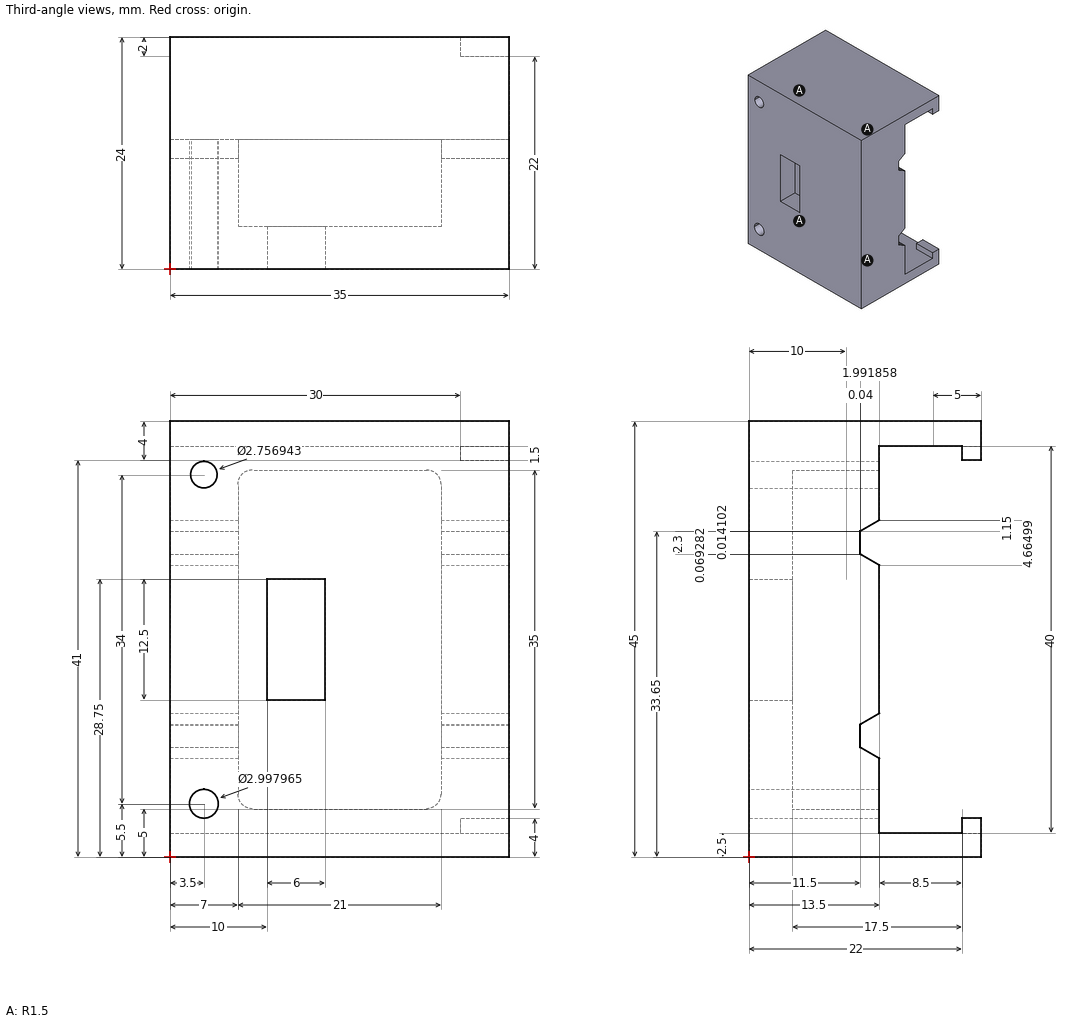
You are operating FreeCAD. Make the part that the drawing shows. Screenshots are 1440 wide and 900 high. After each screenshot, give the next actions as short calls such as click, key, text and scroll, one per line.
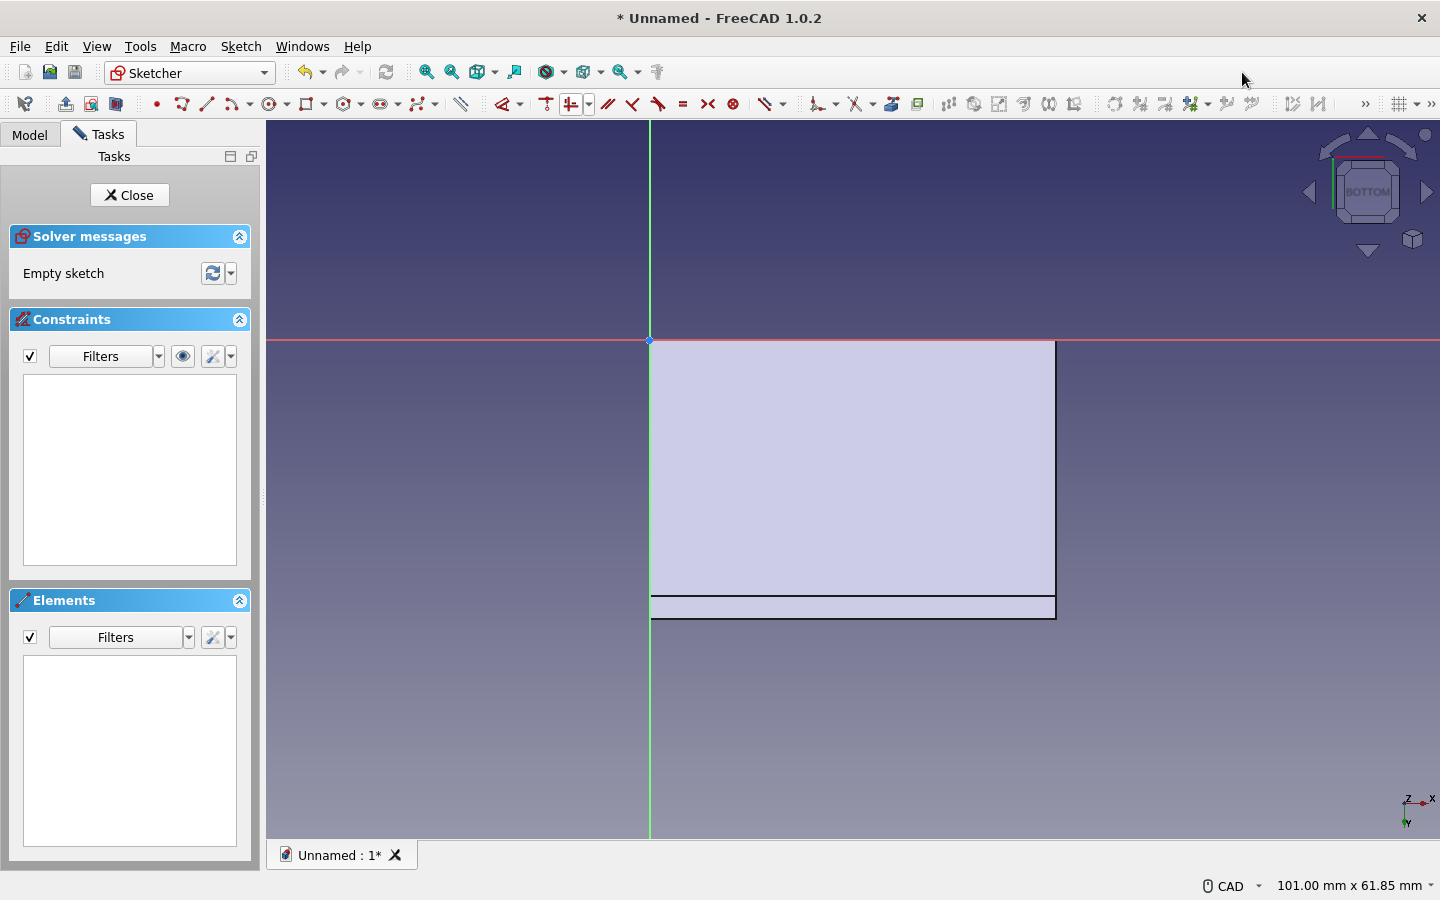
scroll(936, 480, up, 3)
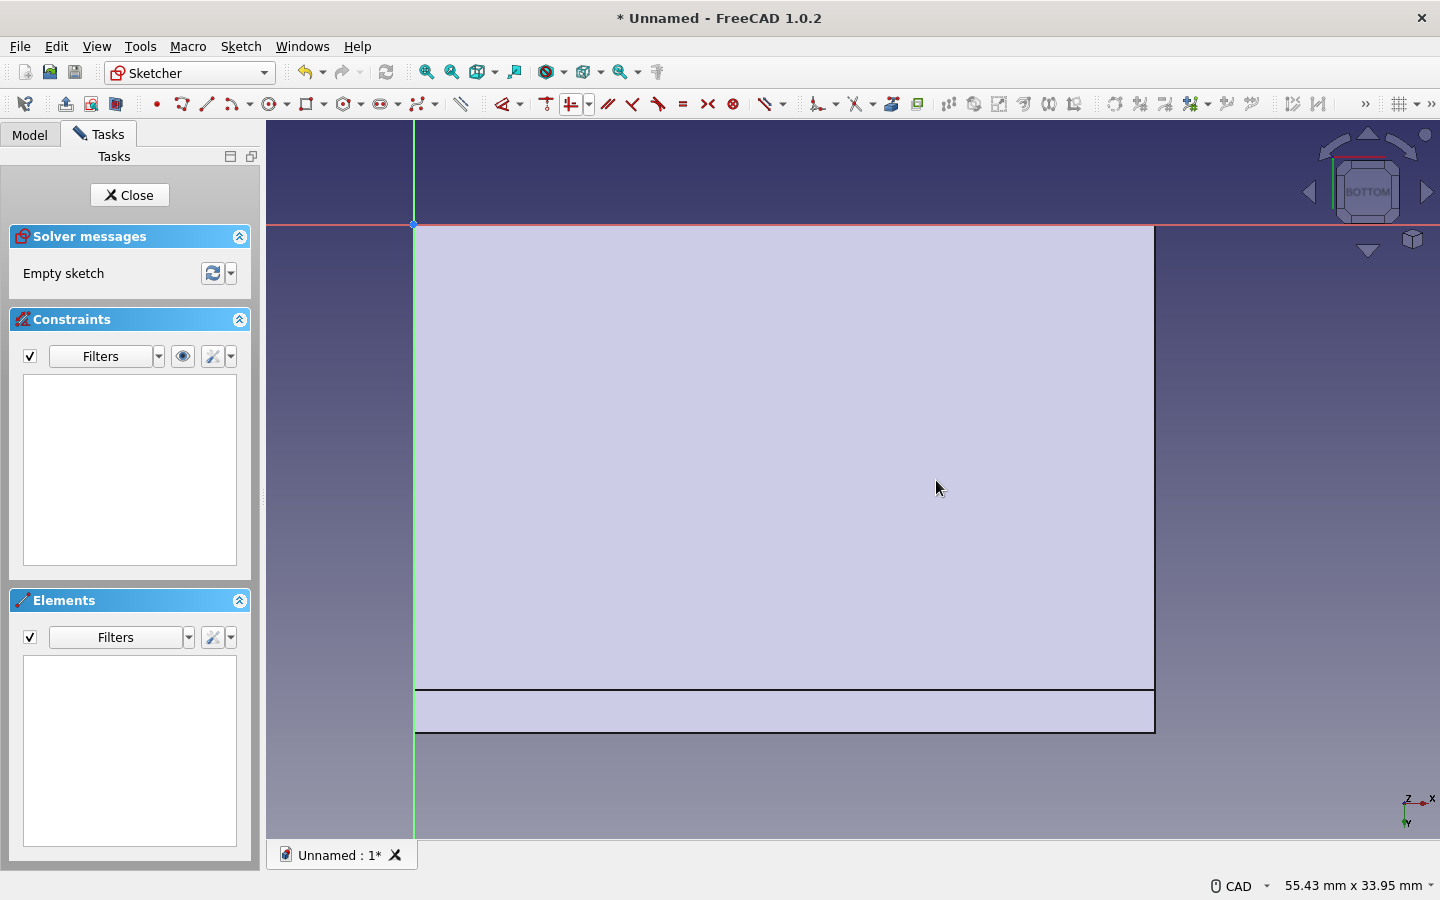
click(306, 104)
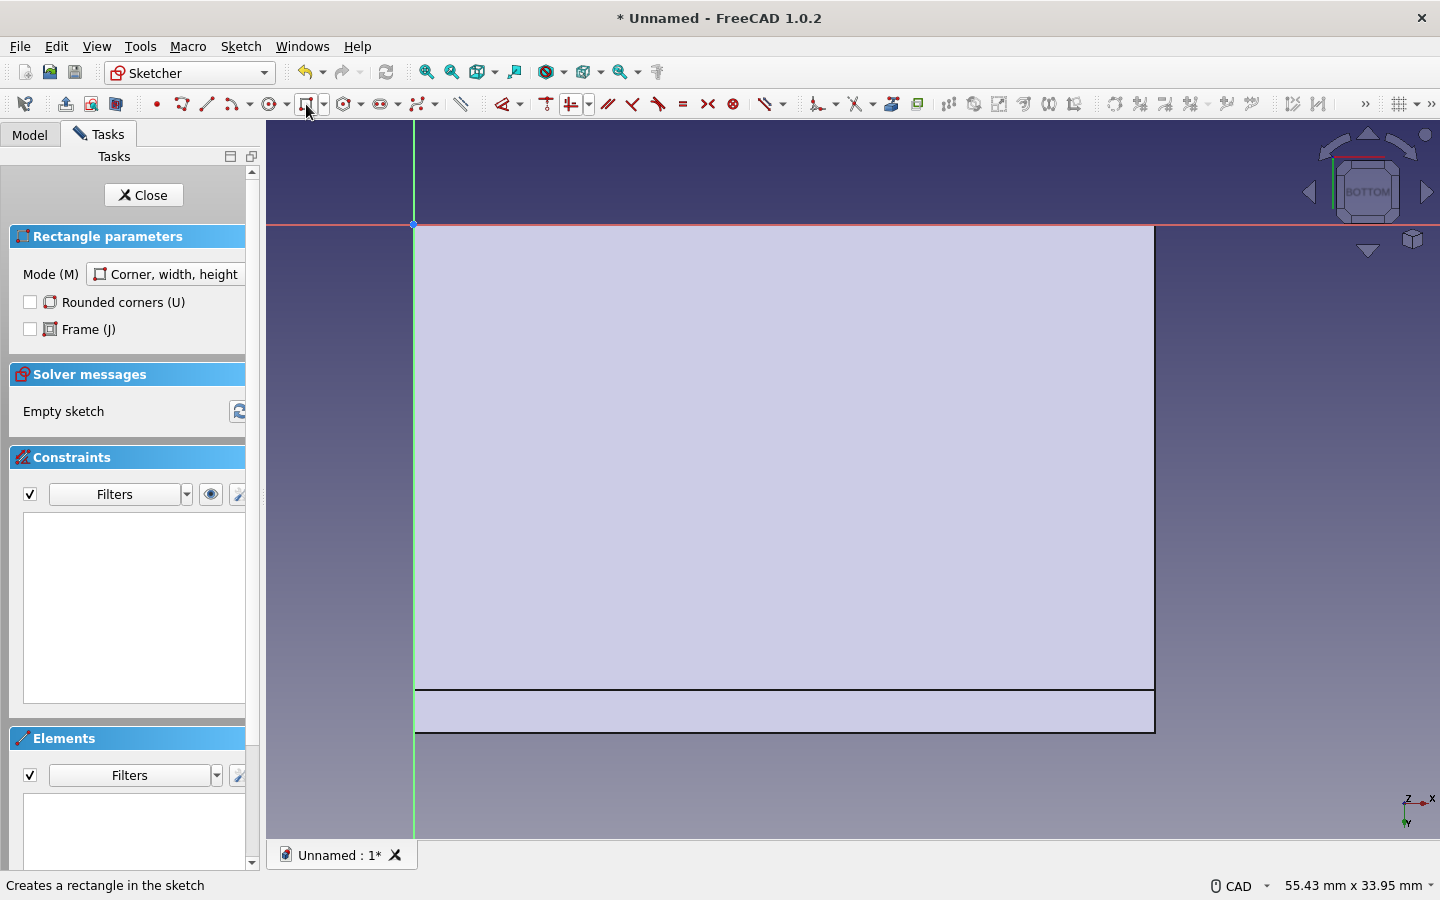
click(414, 690)
click(1155, 733)
key(Escape)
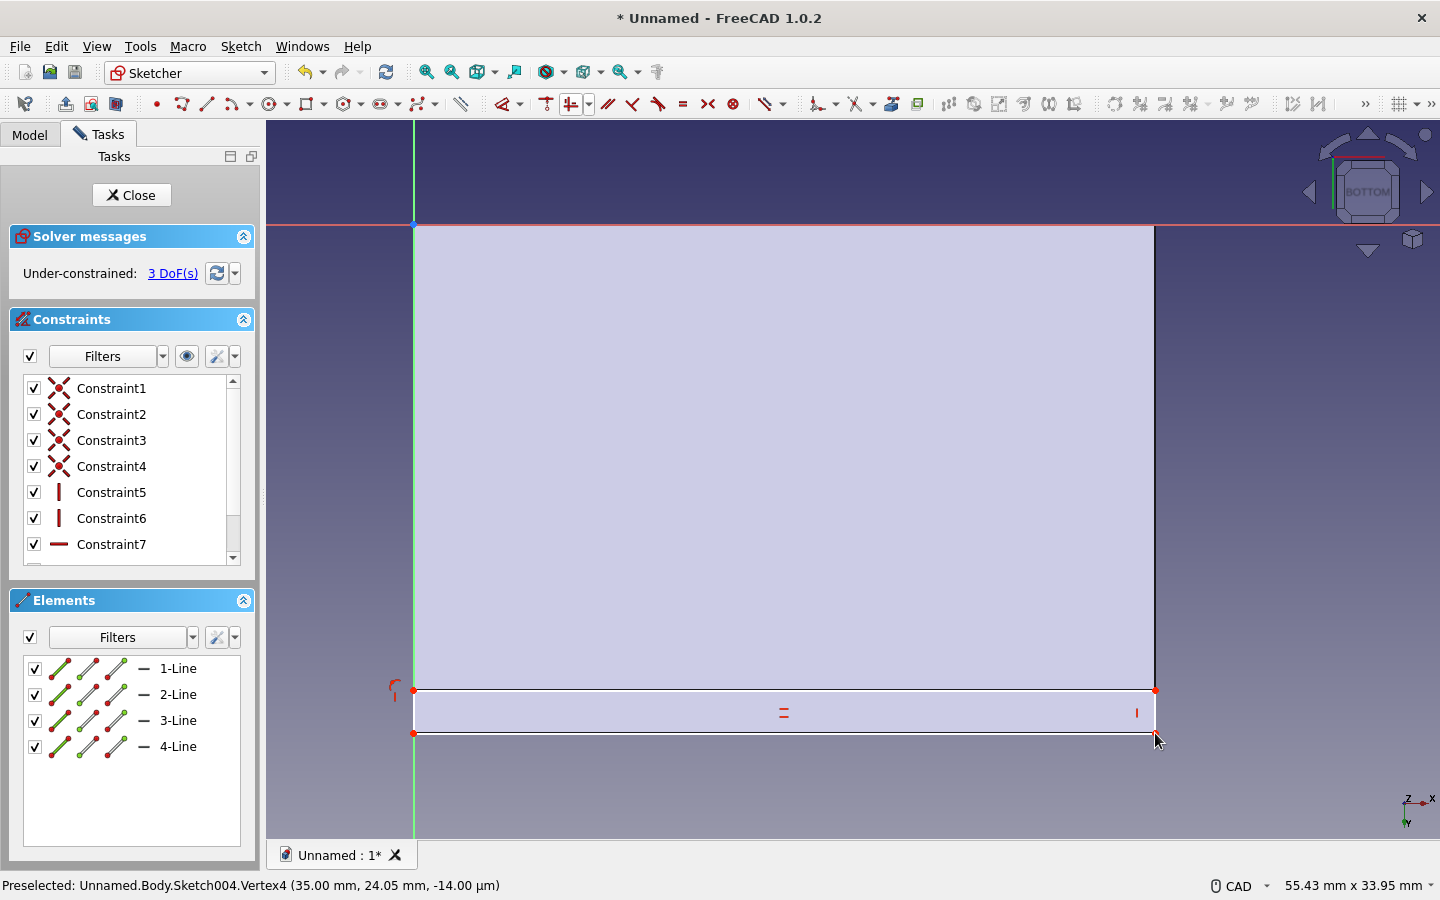
key(d)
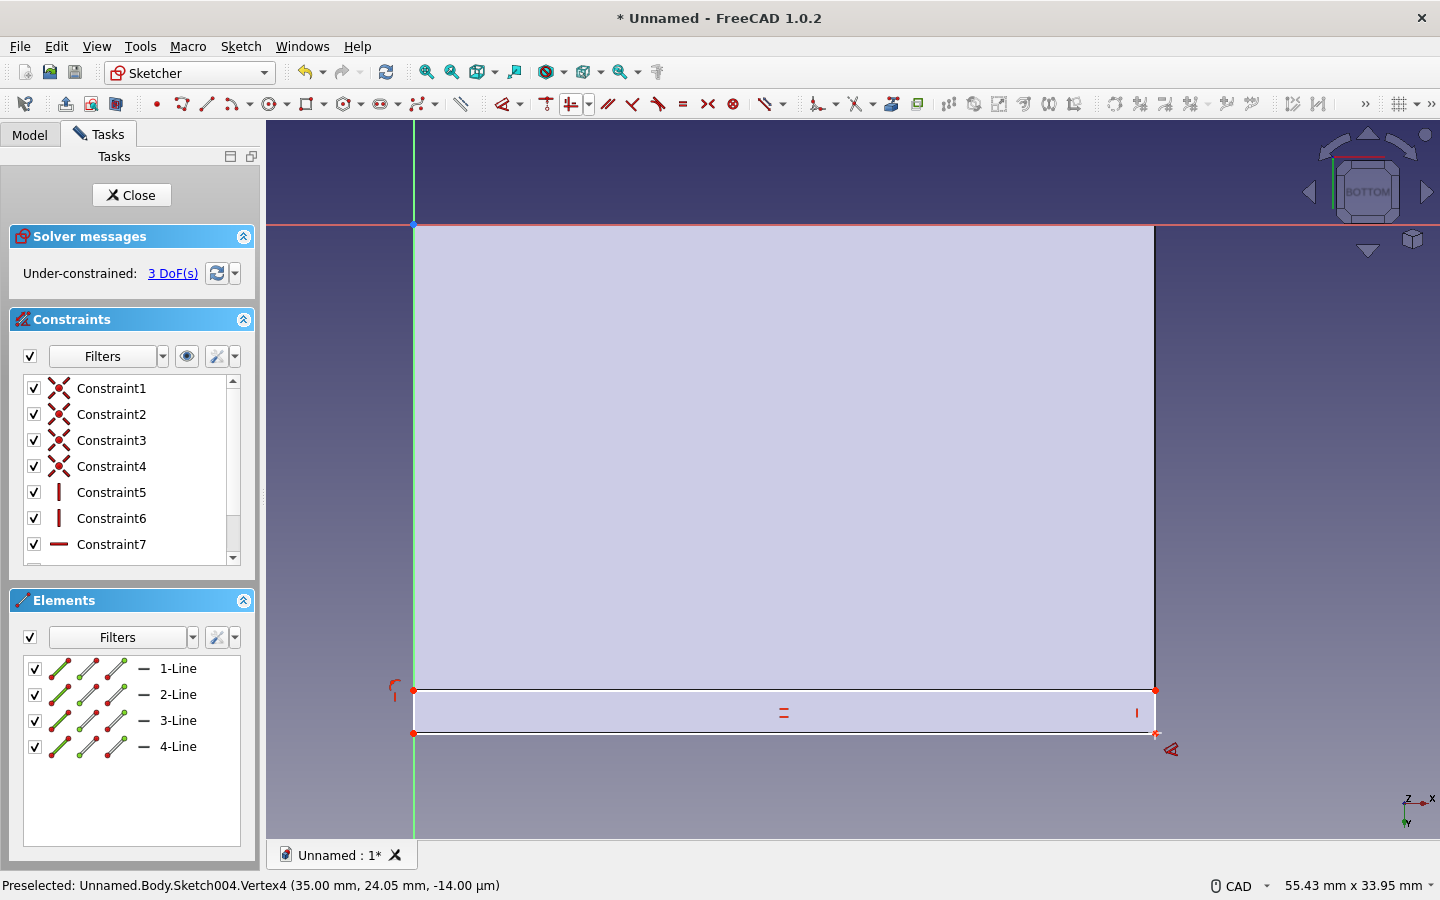
click(414, 704)
click(380, 713)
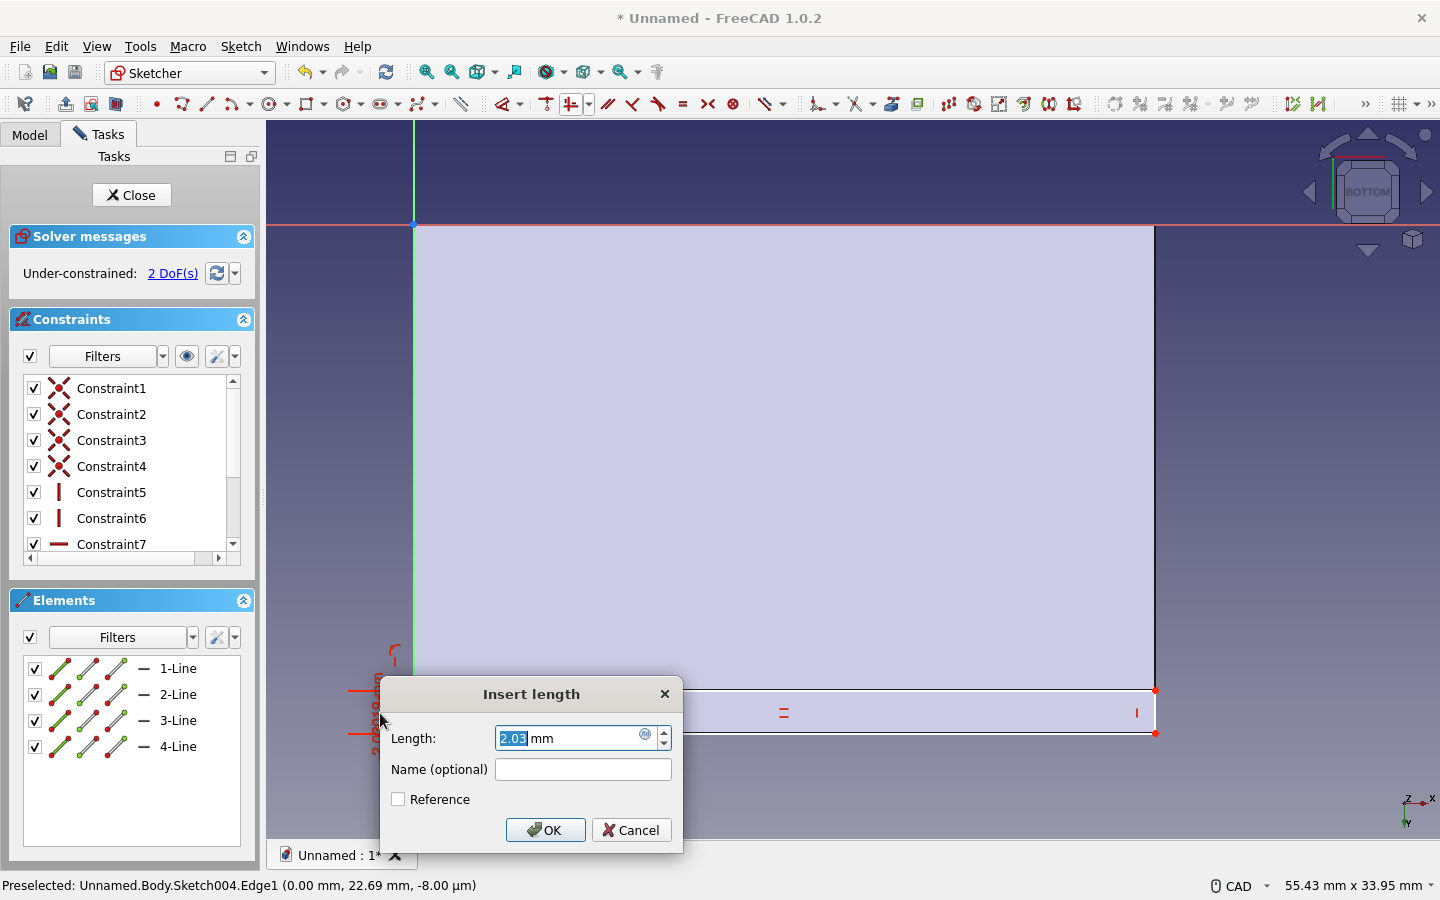
text(2)
key(Return)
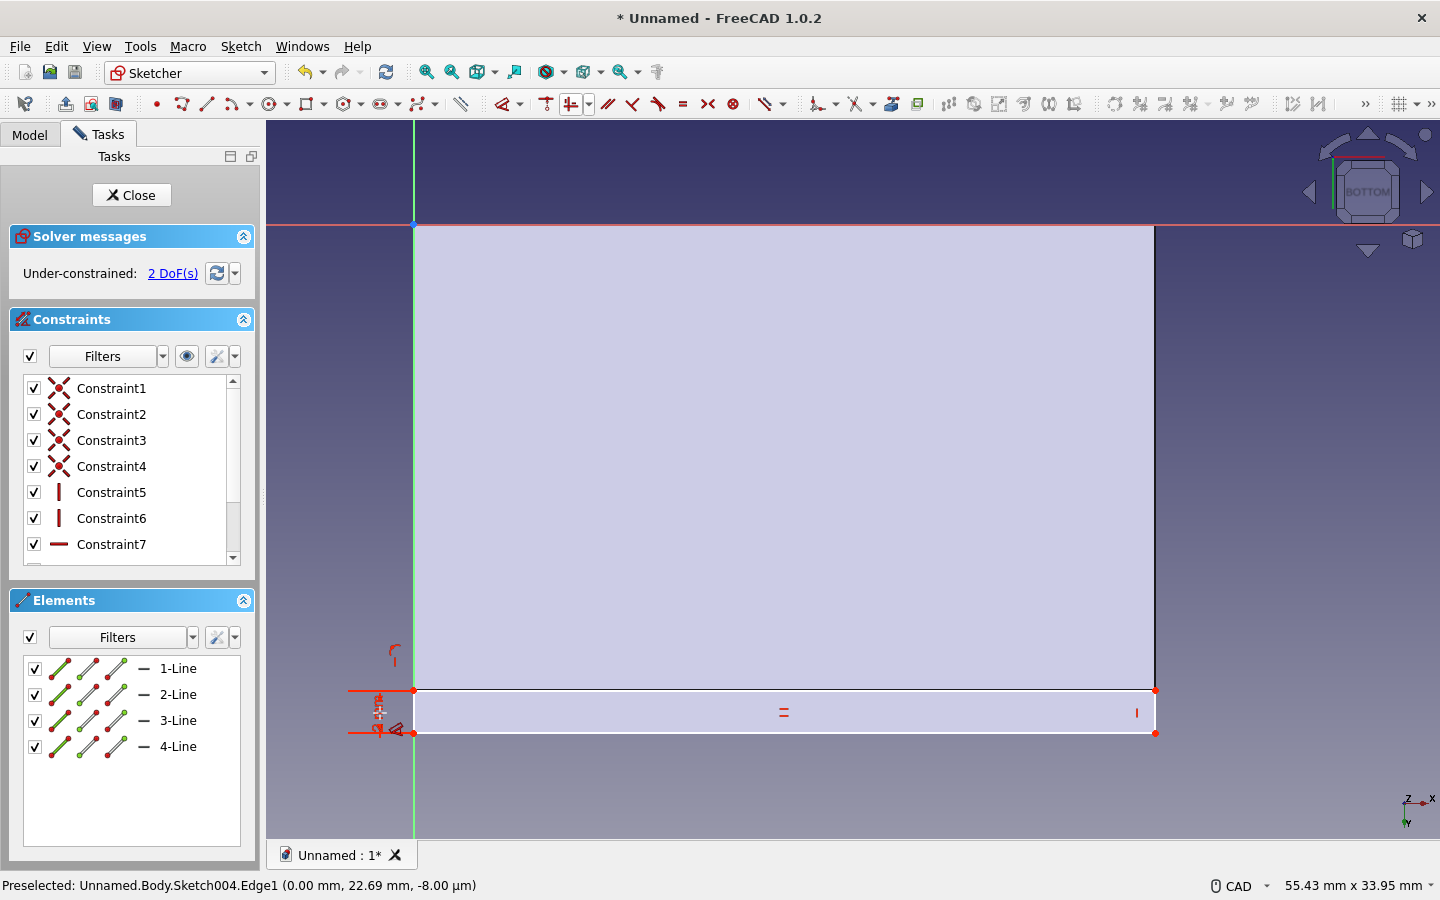
click(636, 733)
click(784, 767)